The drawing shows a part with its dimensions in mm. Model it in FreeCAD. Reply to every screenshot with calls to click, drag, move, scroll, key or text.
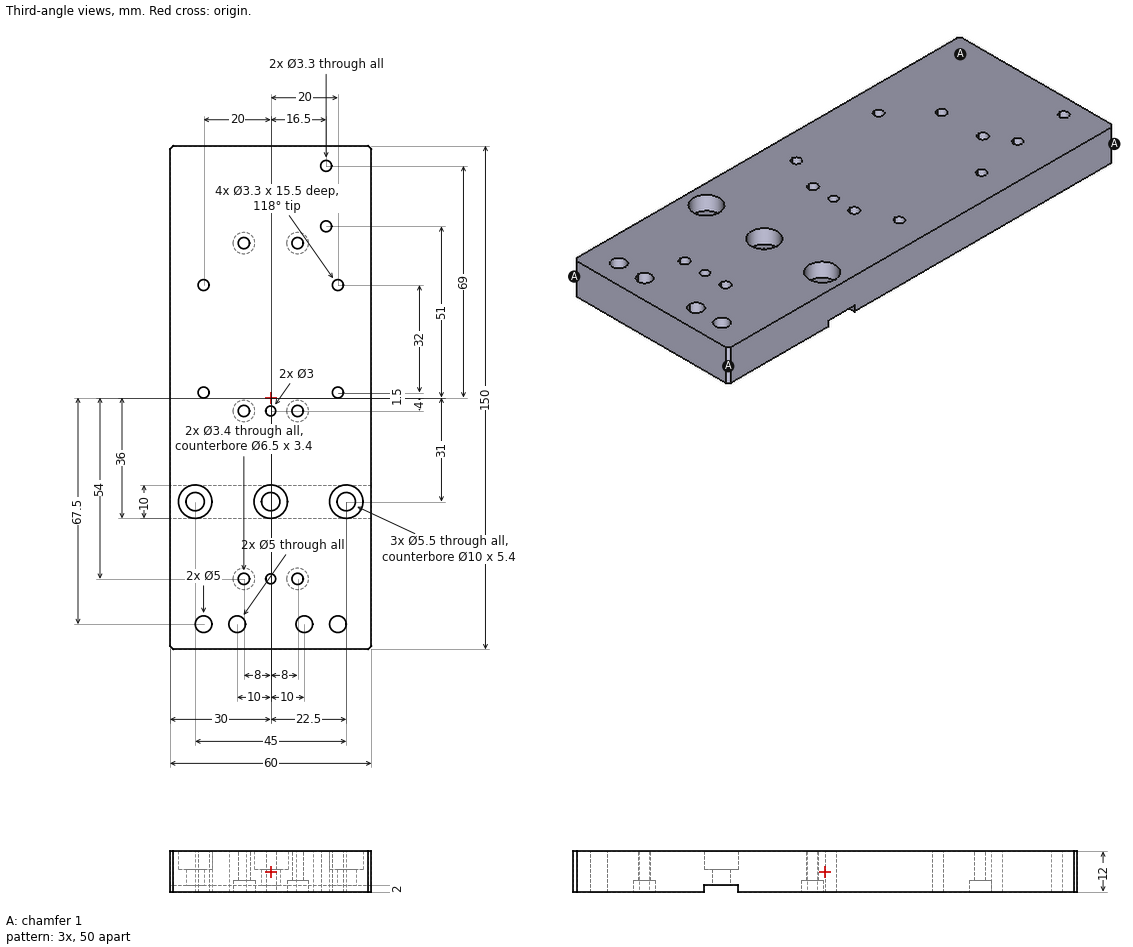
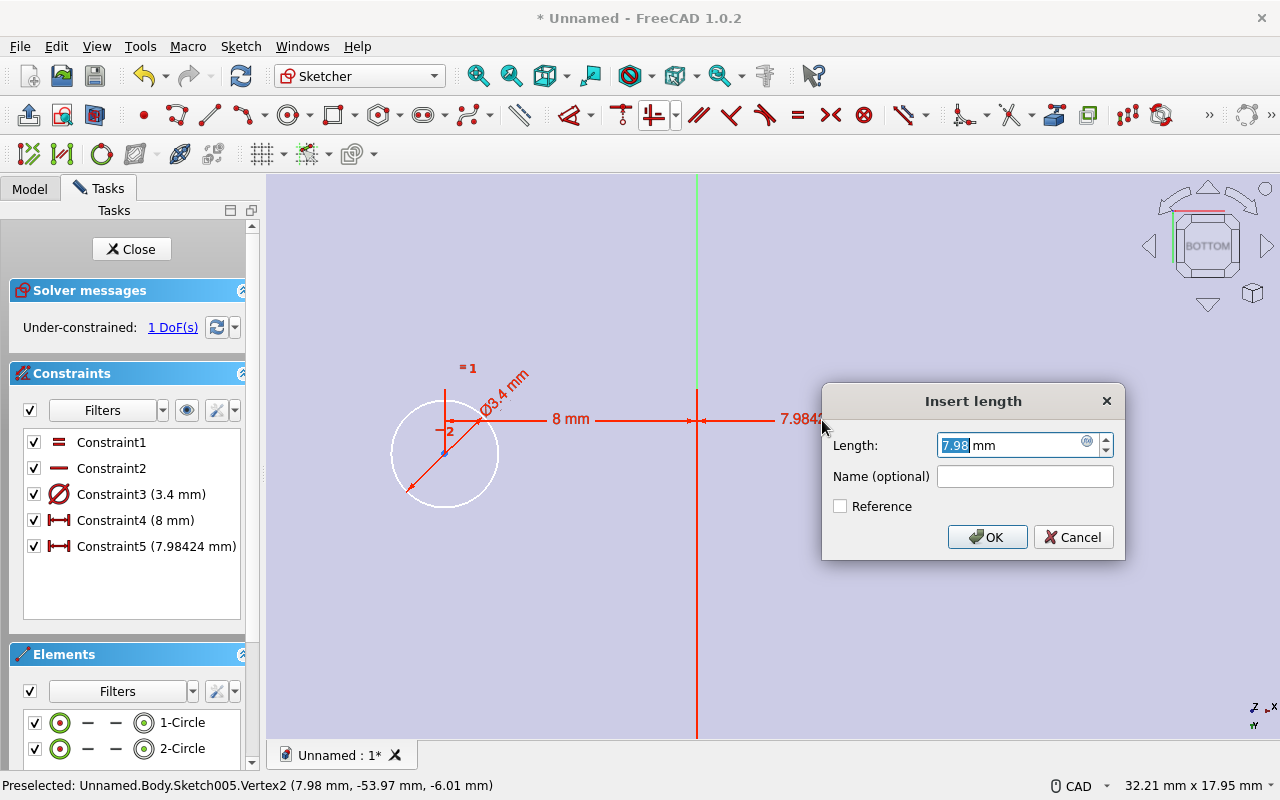
text(8)
key(Return)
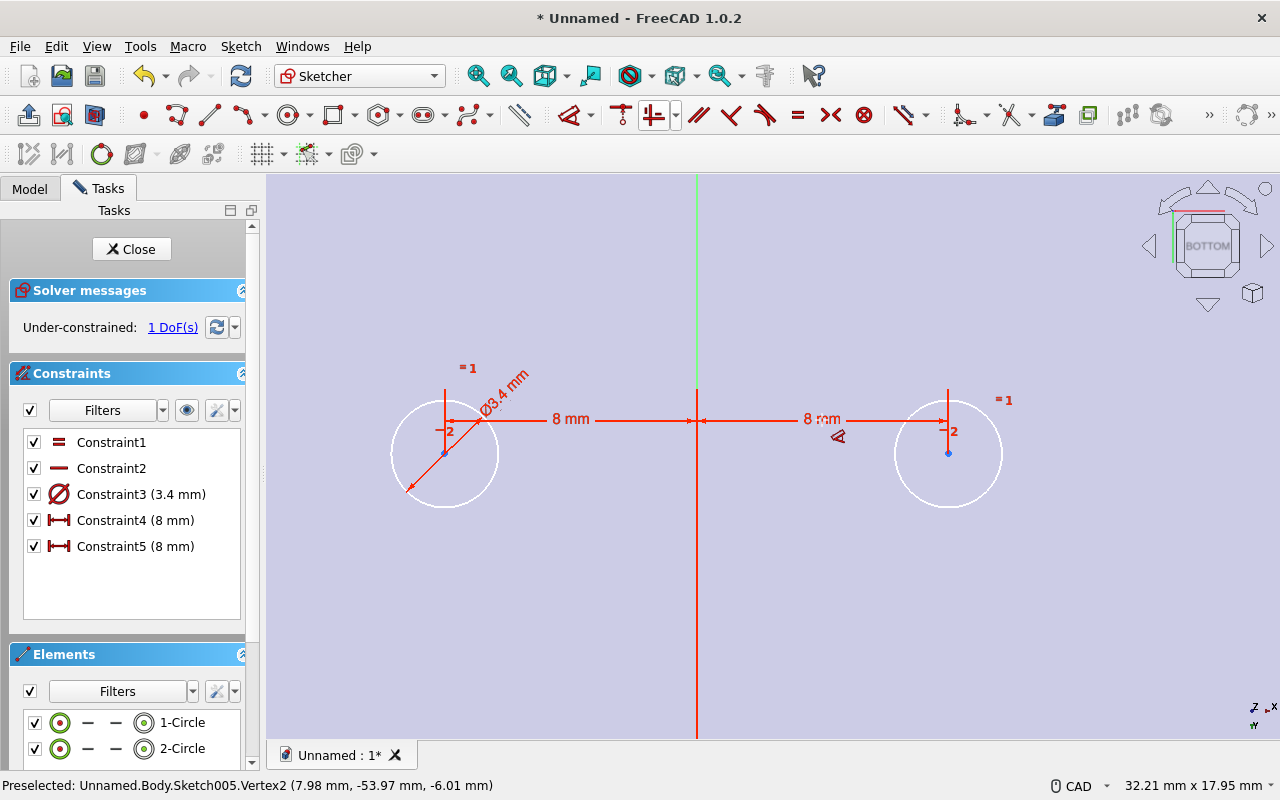
click(445, 454)
click(411, 582)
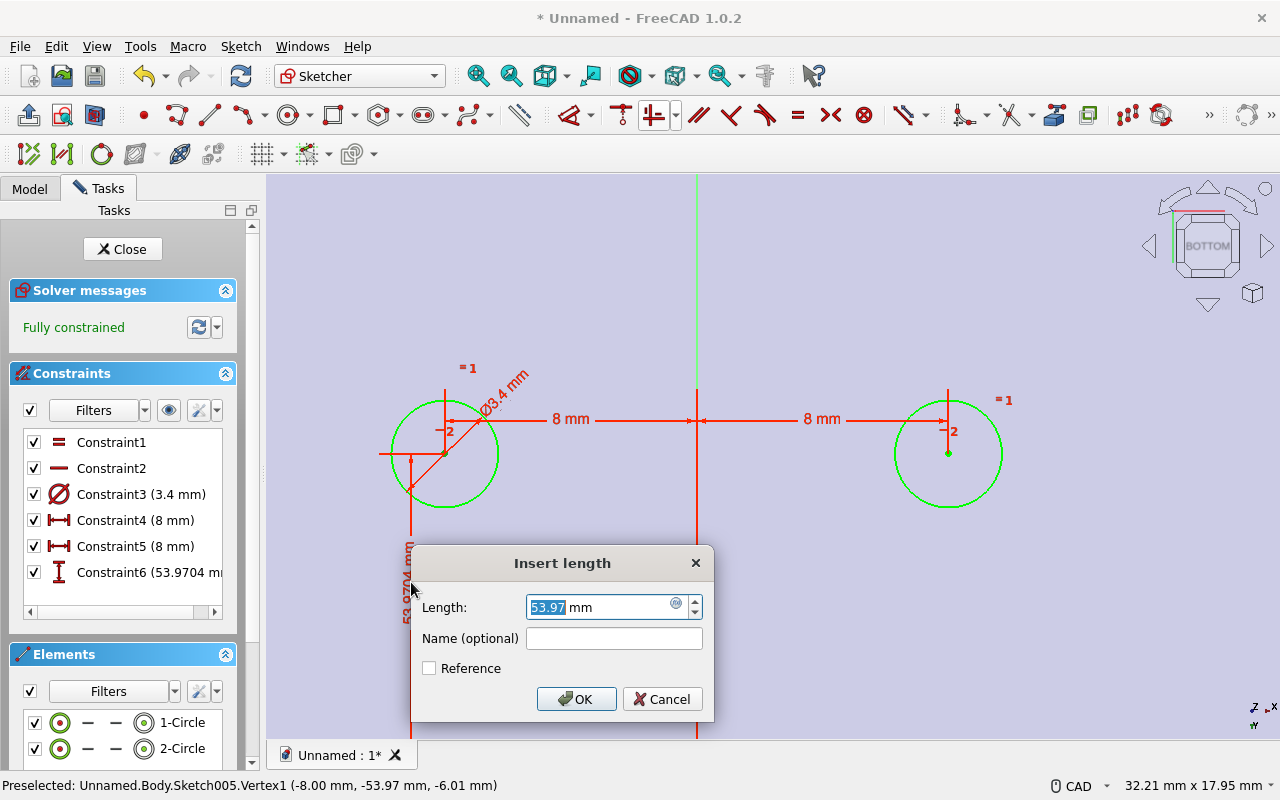
text(54)
key(Return)
key(Escape)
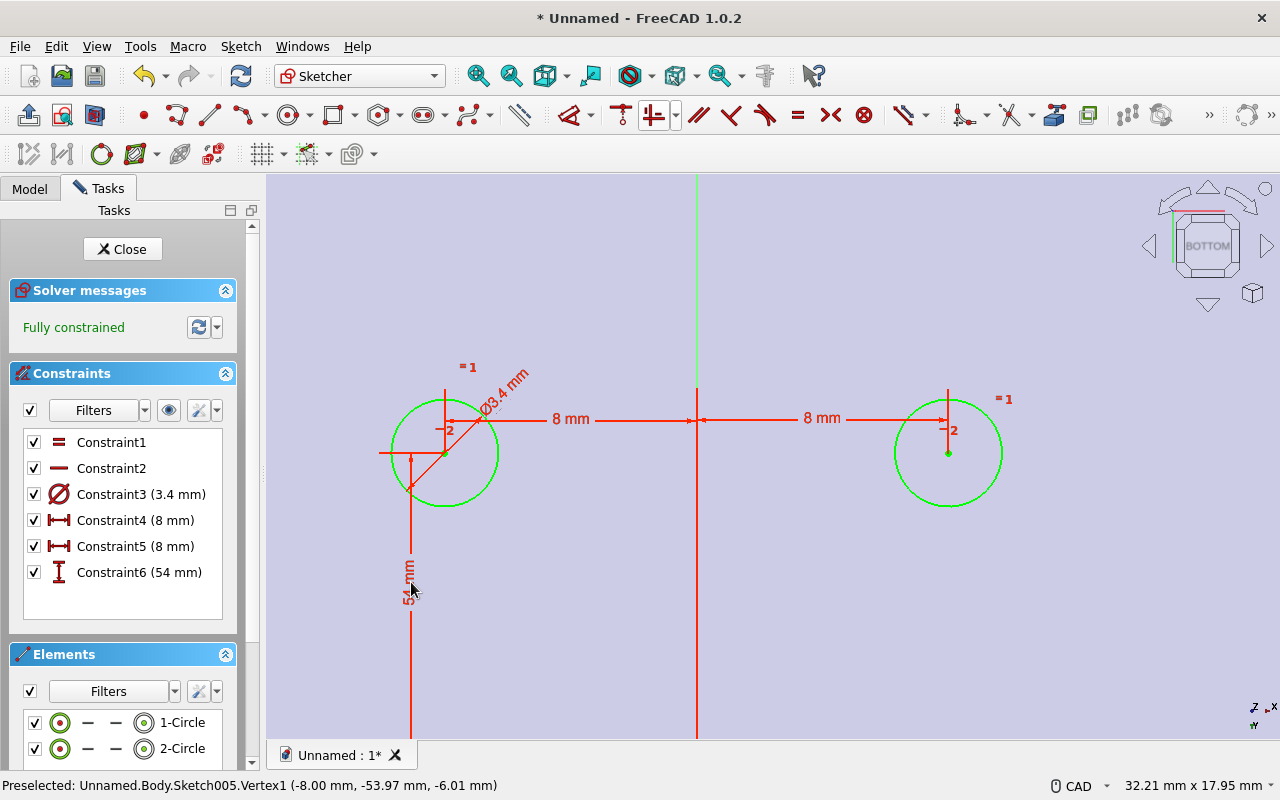
click(123, 249)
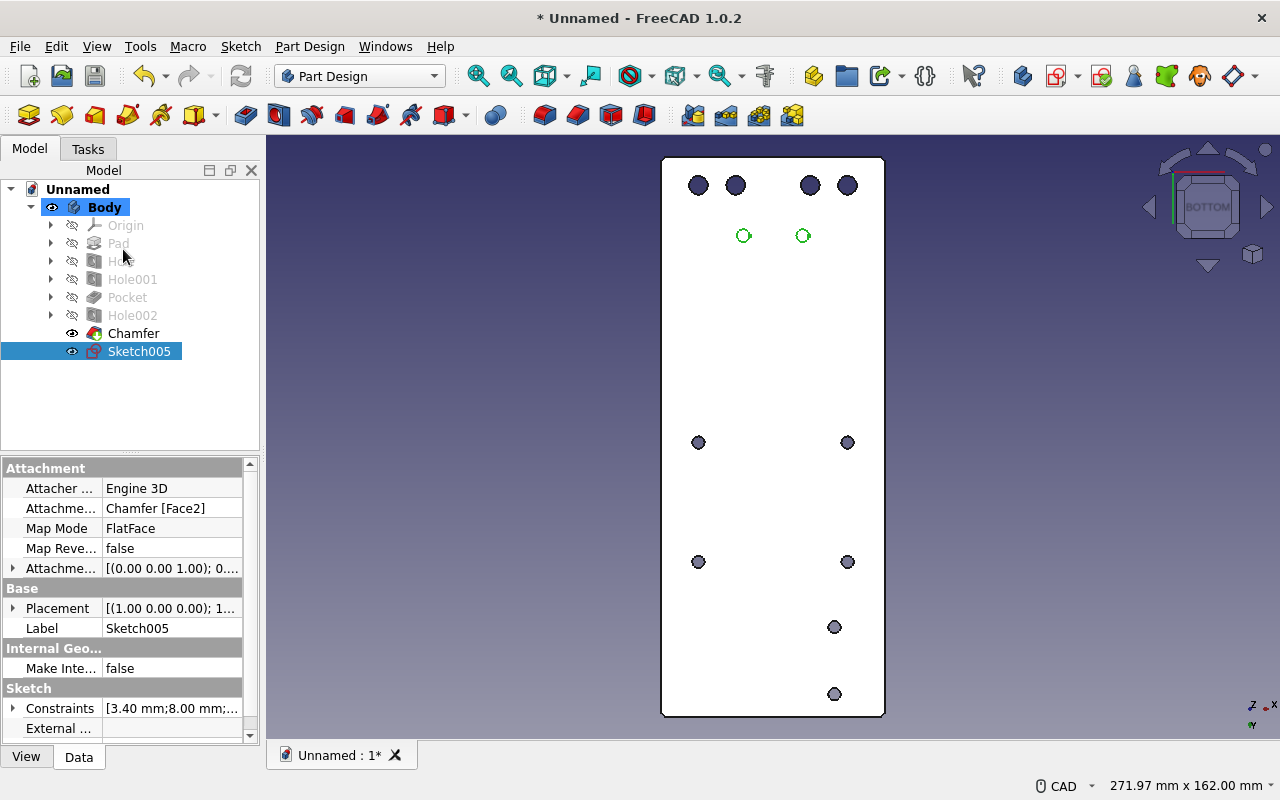
click(279, 116)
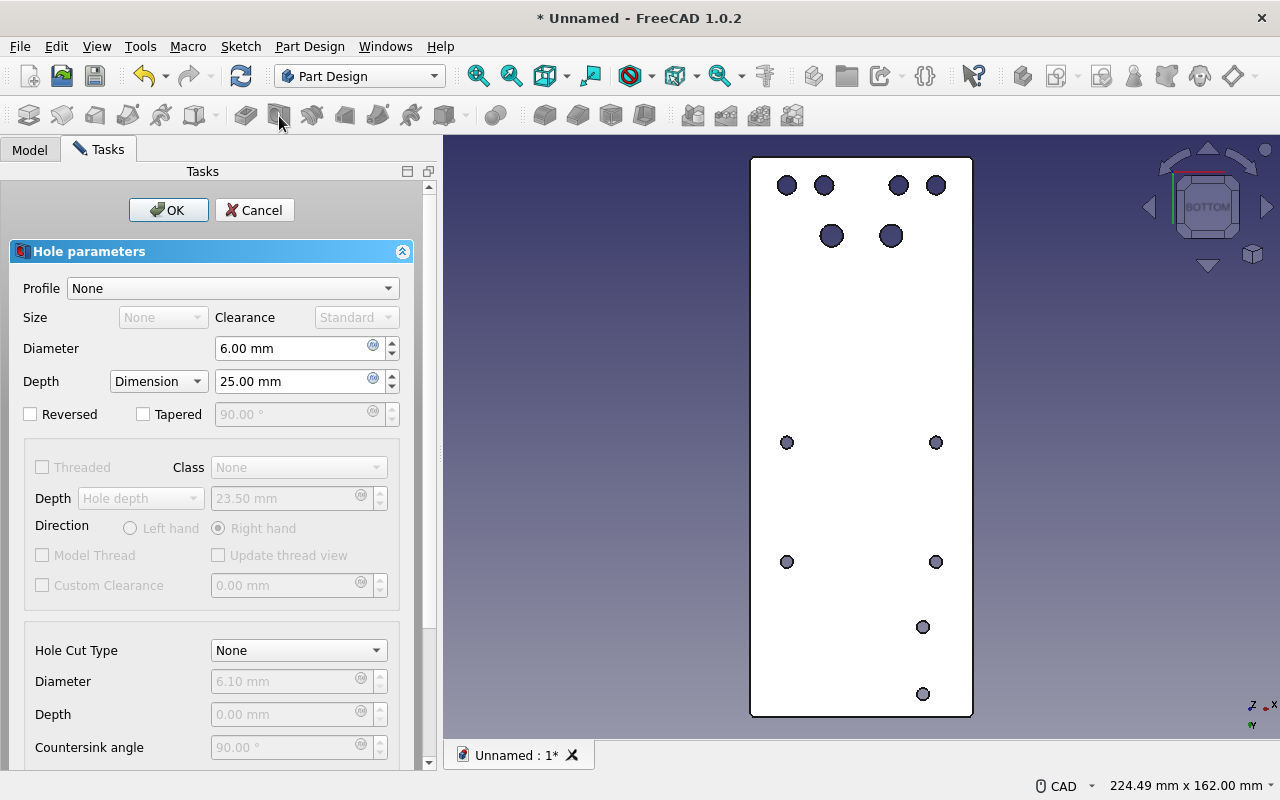
triple_click(300, 348)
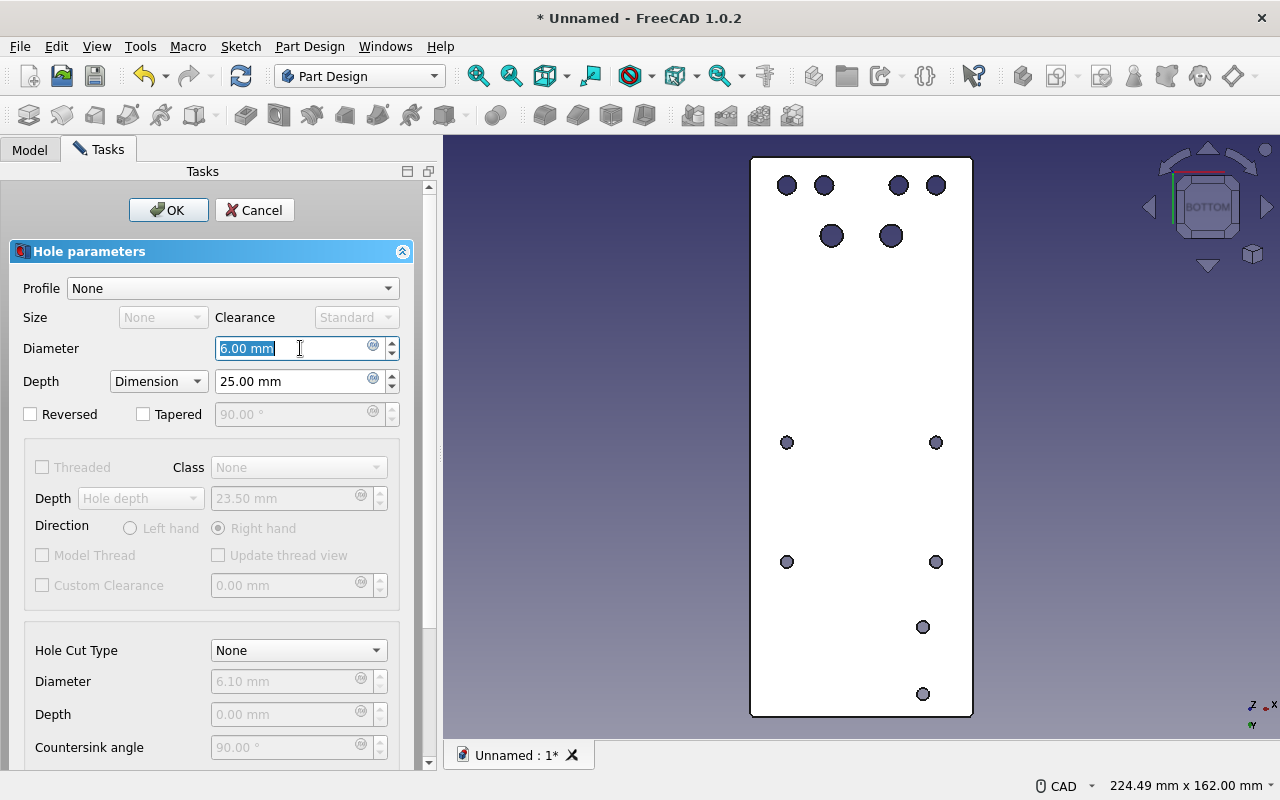
text(3.4)
key(Tab)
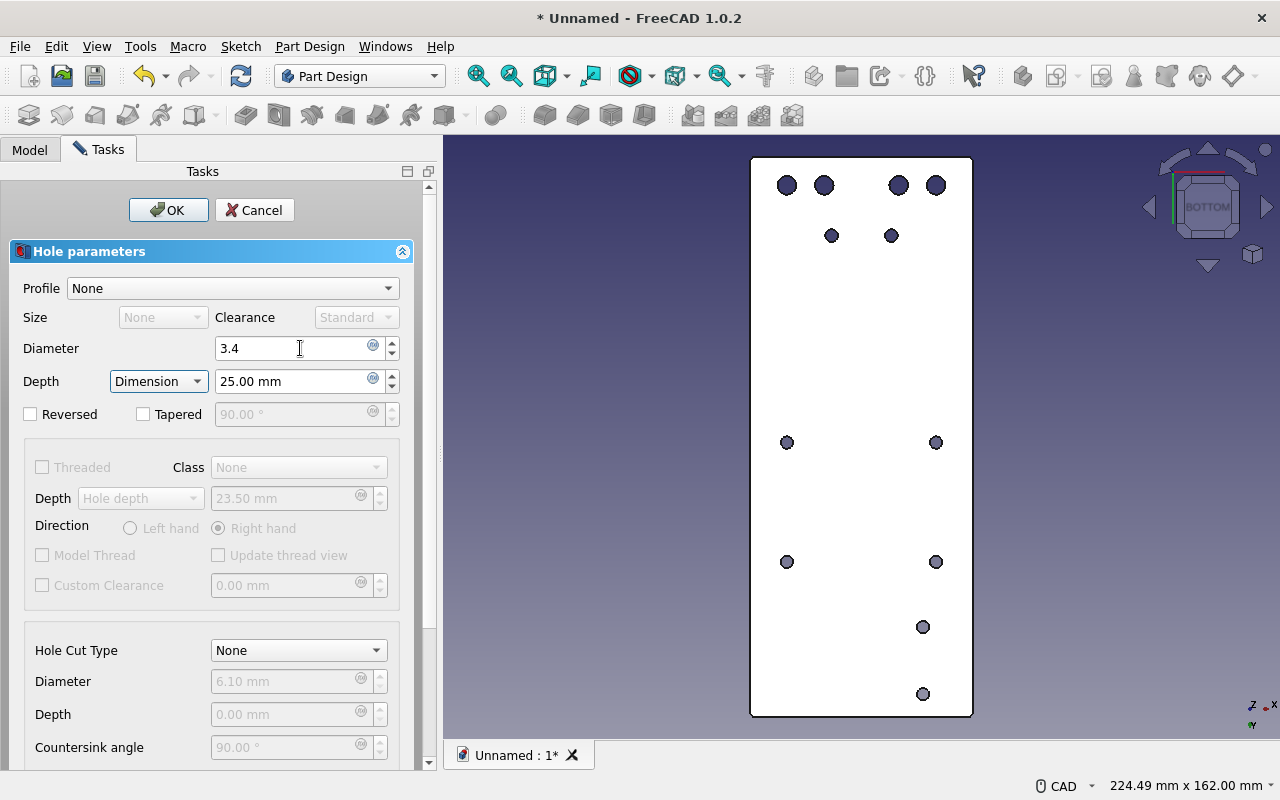
click(160, 382)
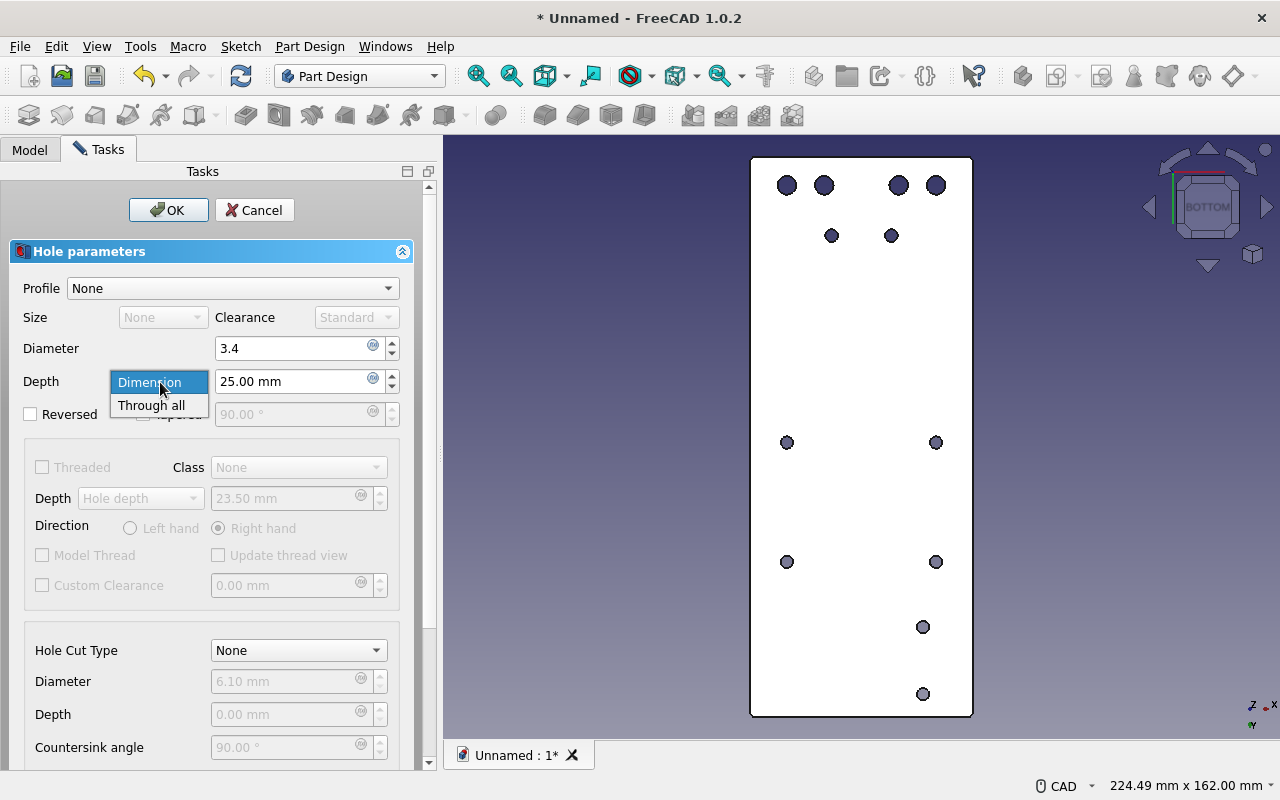
click(158, 406)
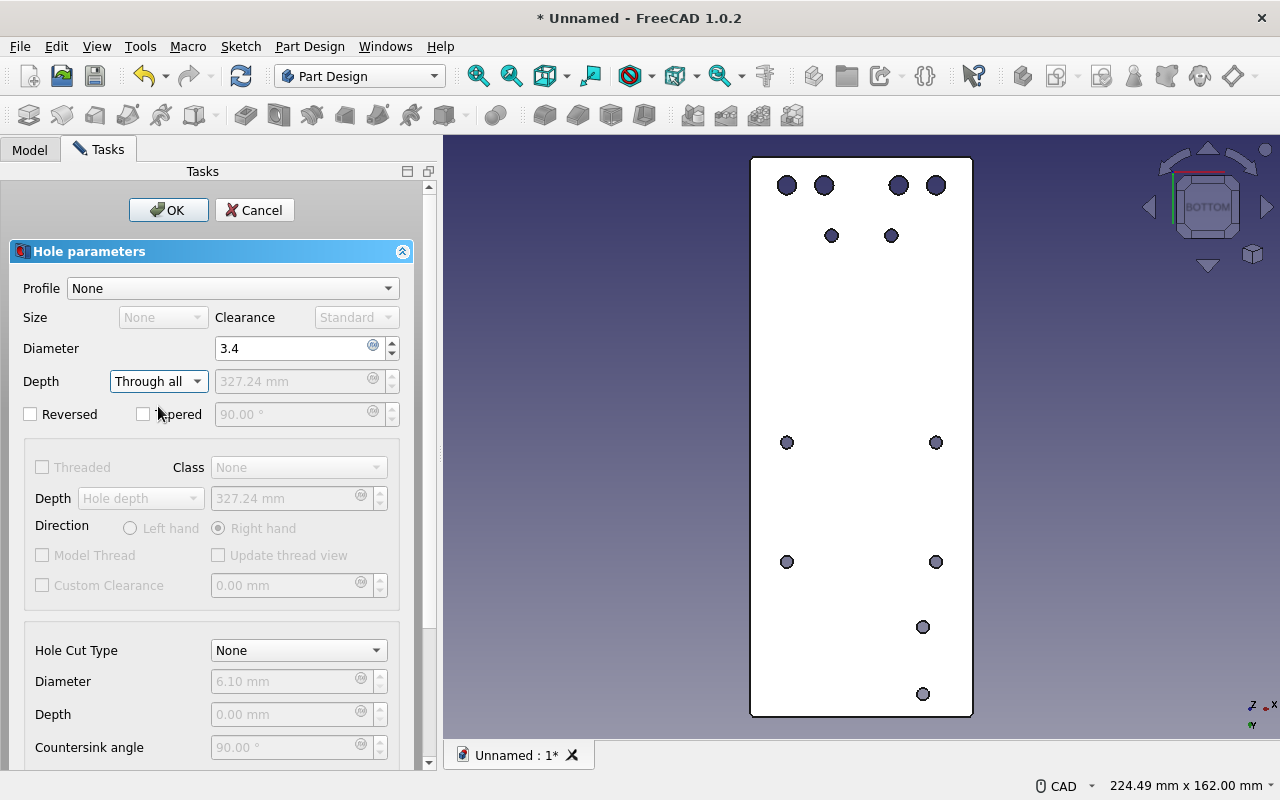
click(300, 650)